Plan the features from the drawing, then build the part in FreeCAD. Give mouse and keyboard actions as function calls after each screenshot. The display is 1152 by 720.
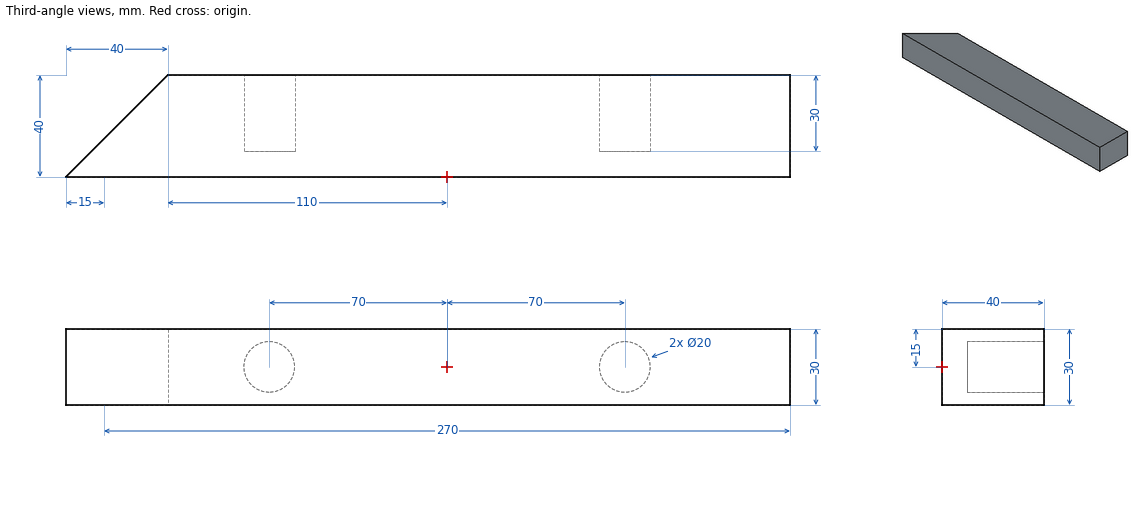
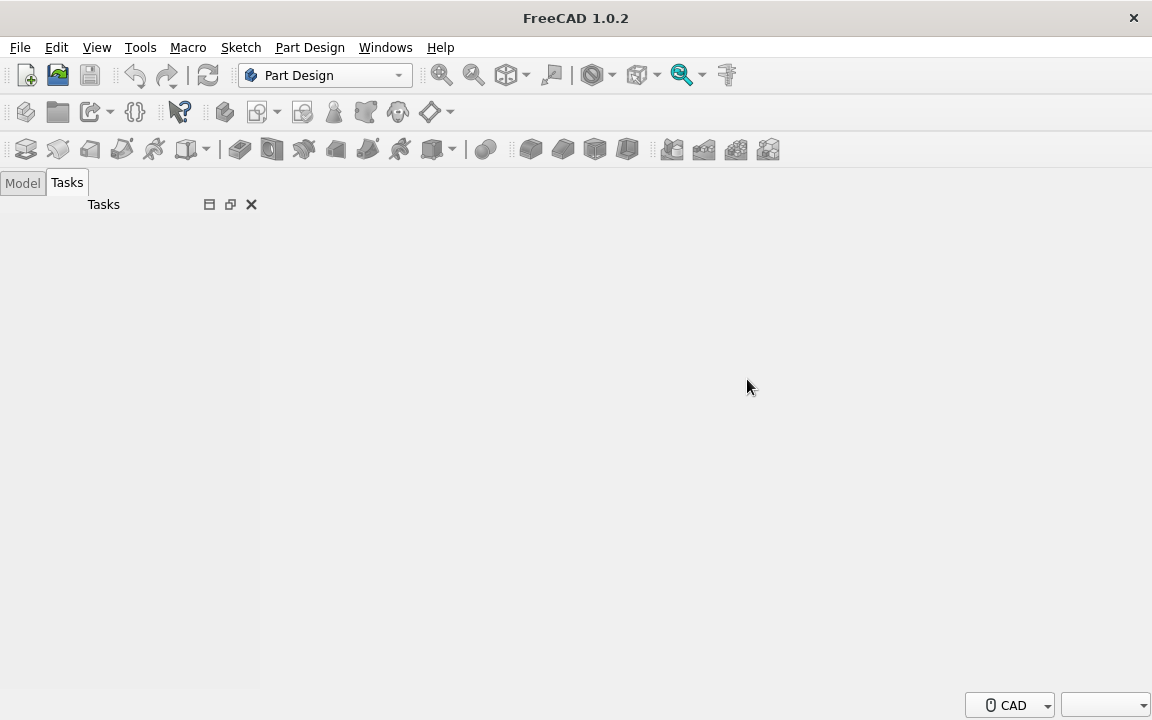
key(ctrl+n)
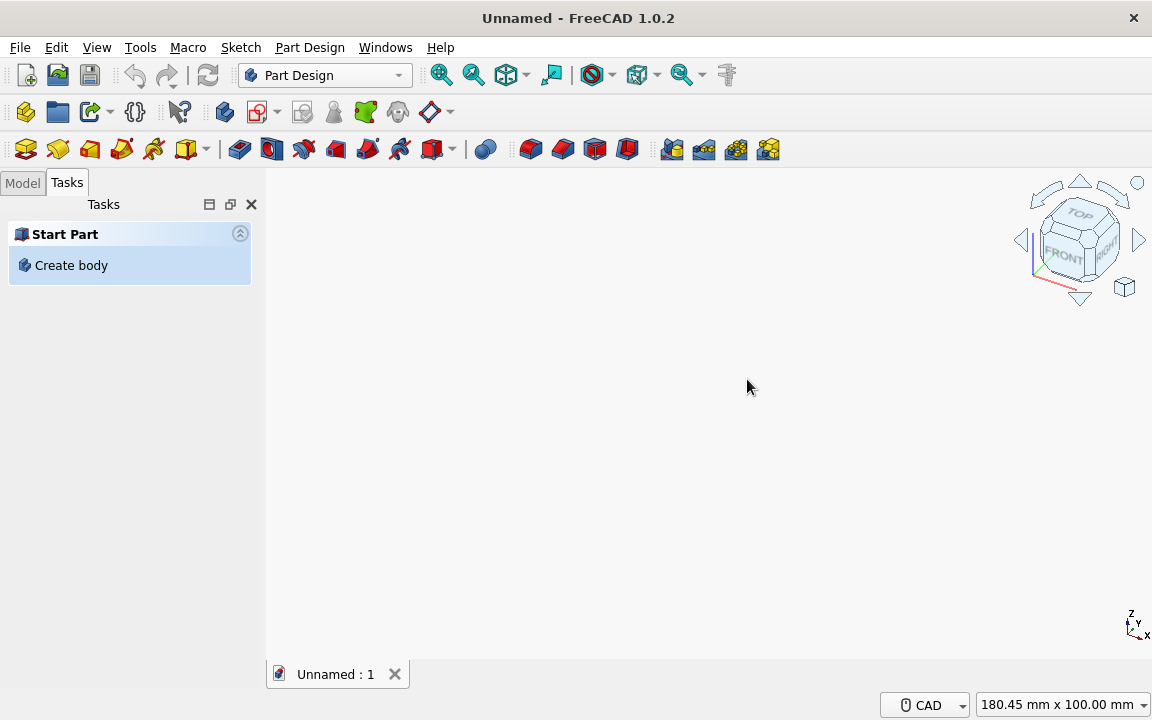
click(258, 112)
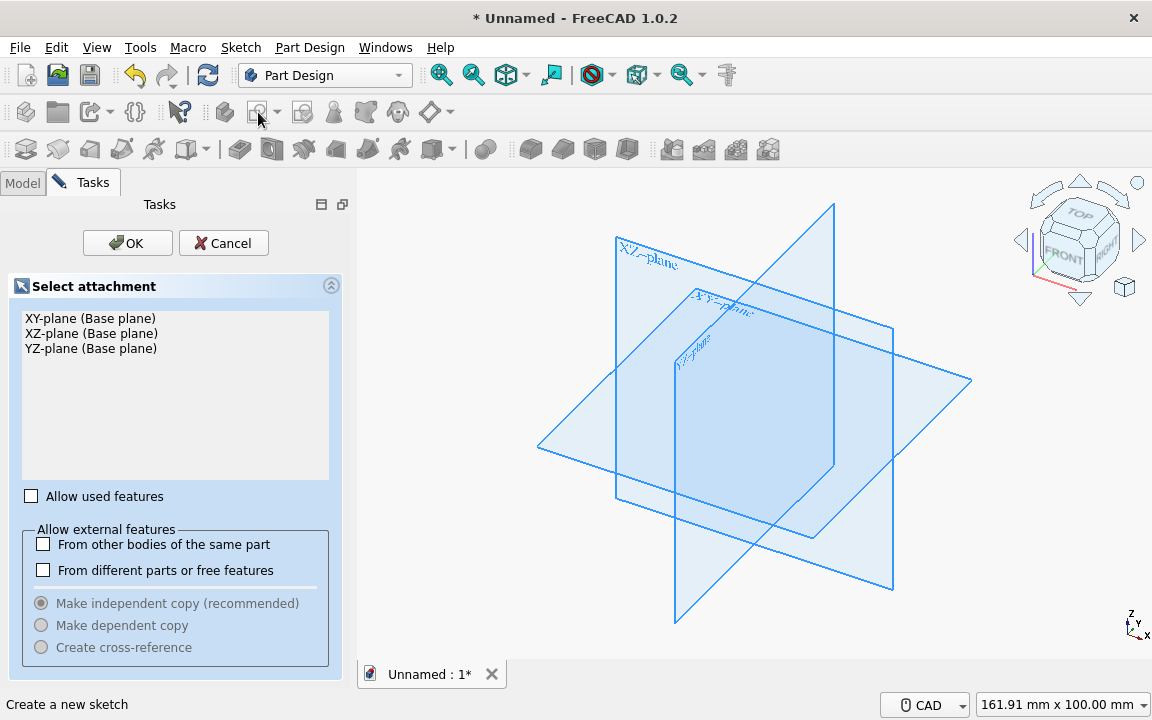
click(82, 334)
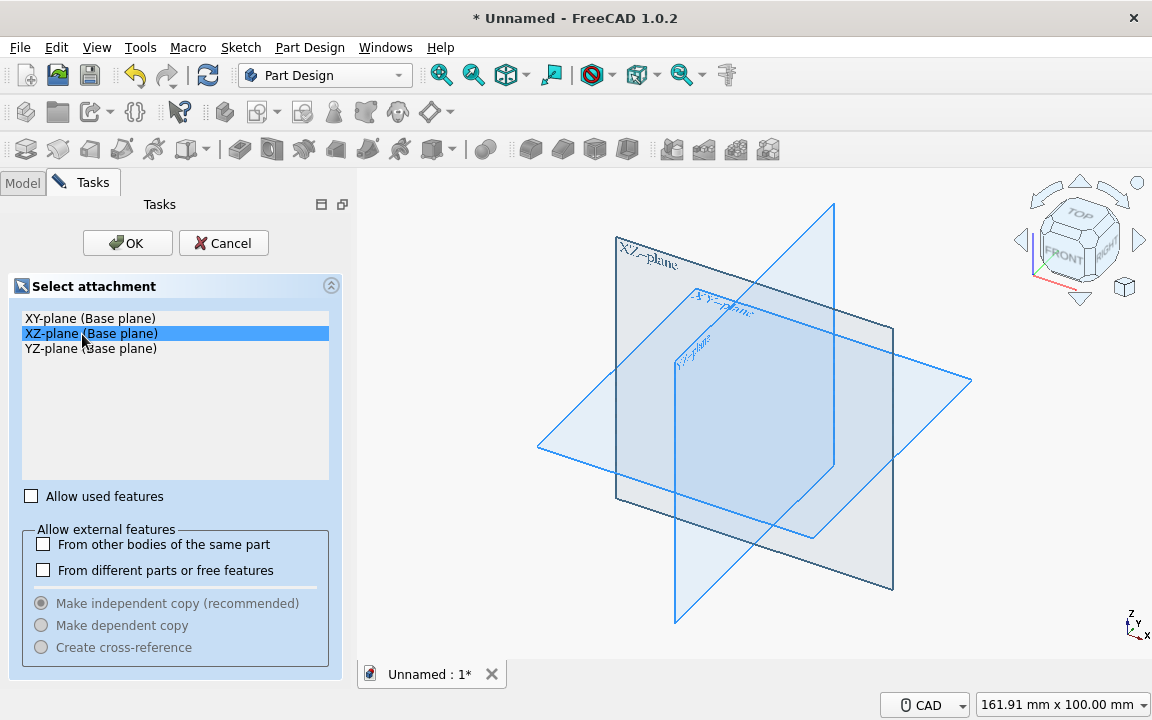
click(128, 243)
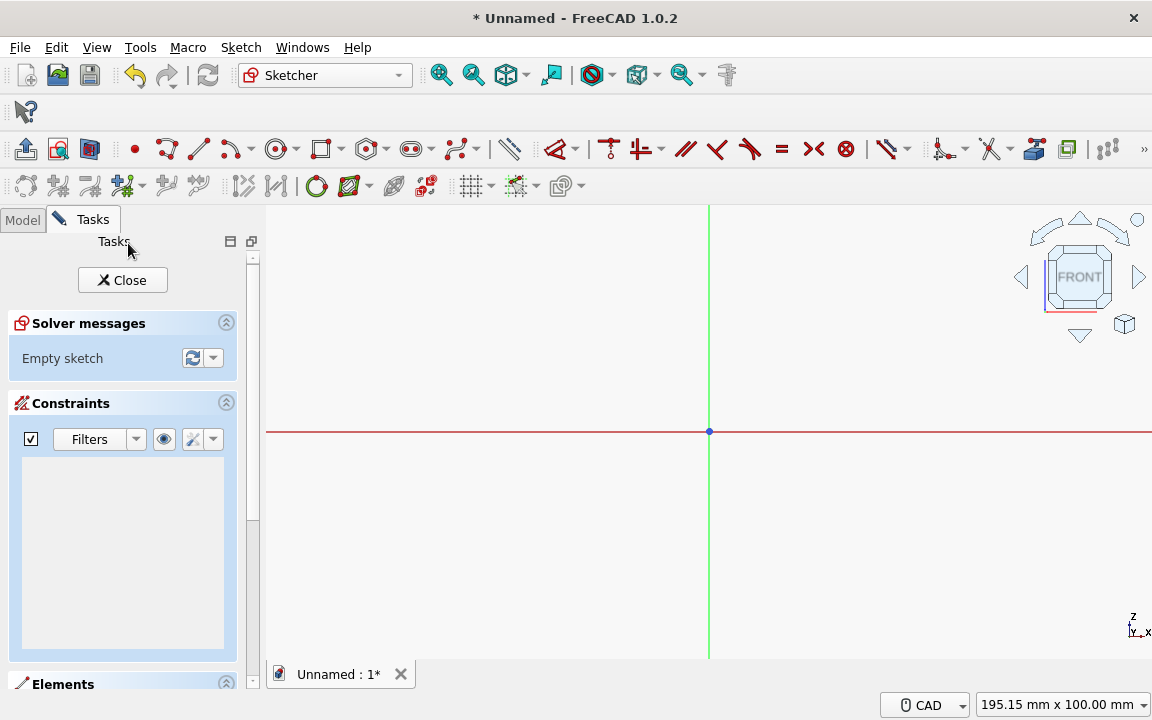
scroll(601, 432, down, 5)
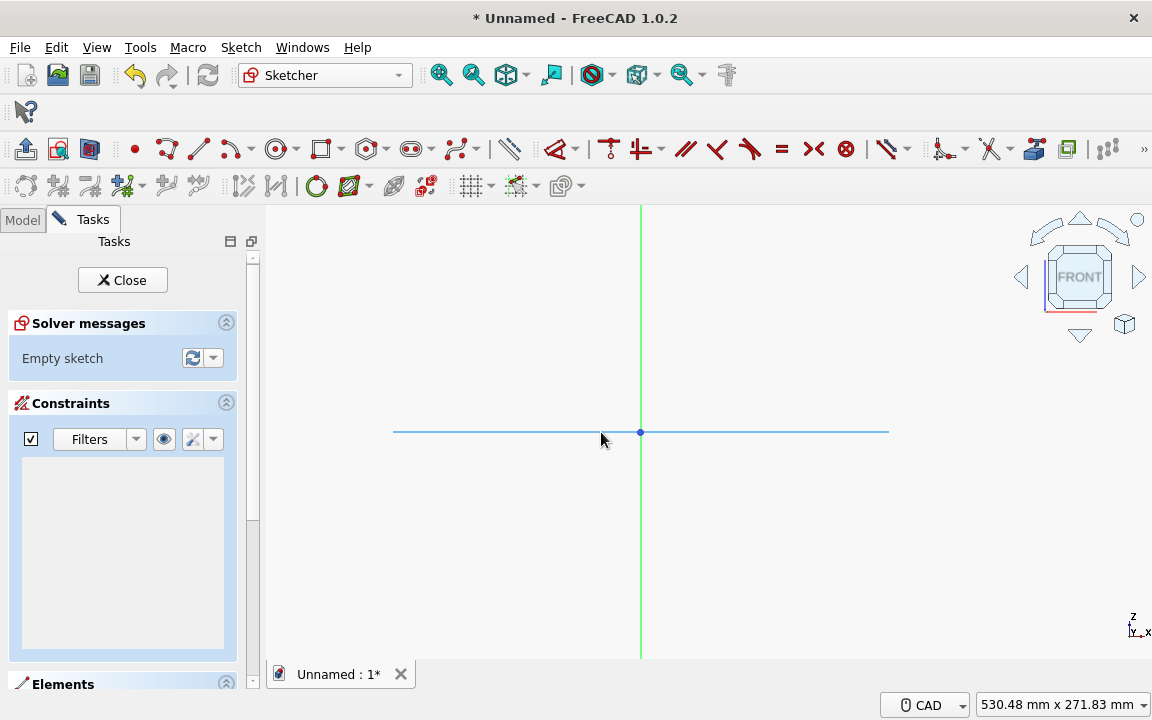
key(g)
key(v)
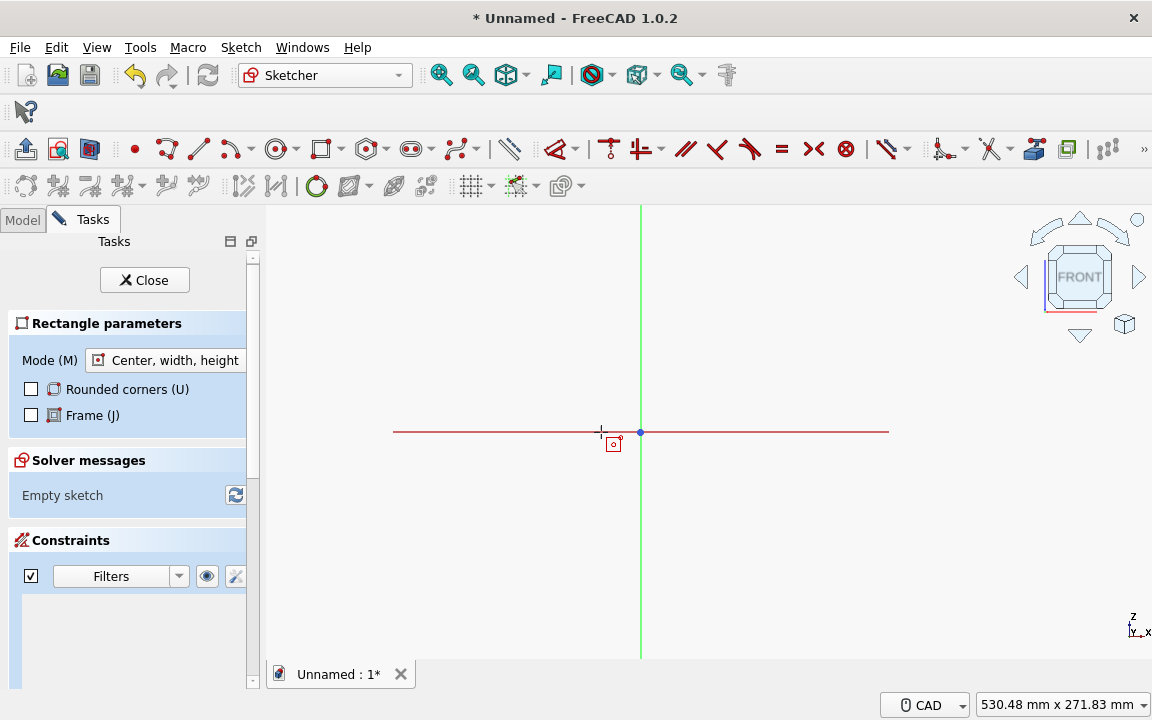
click(641, 432)
move(866, 407)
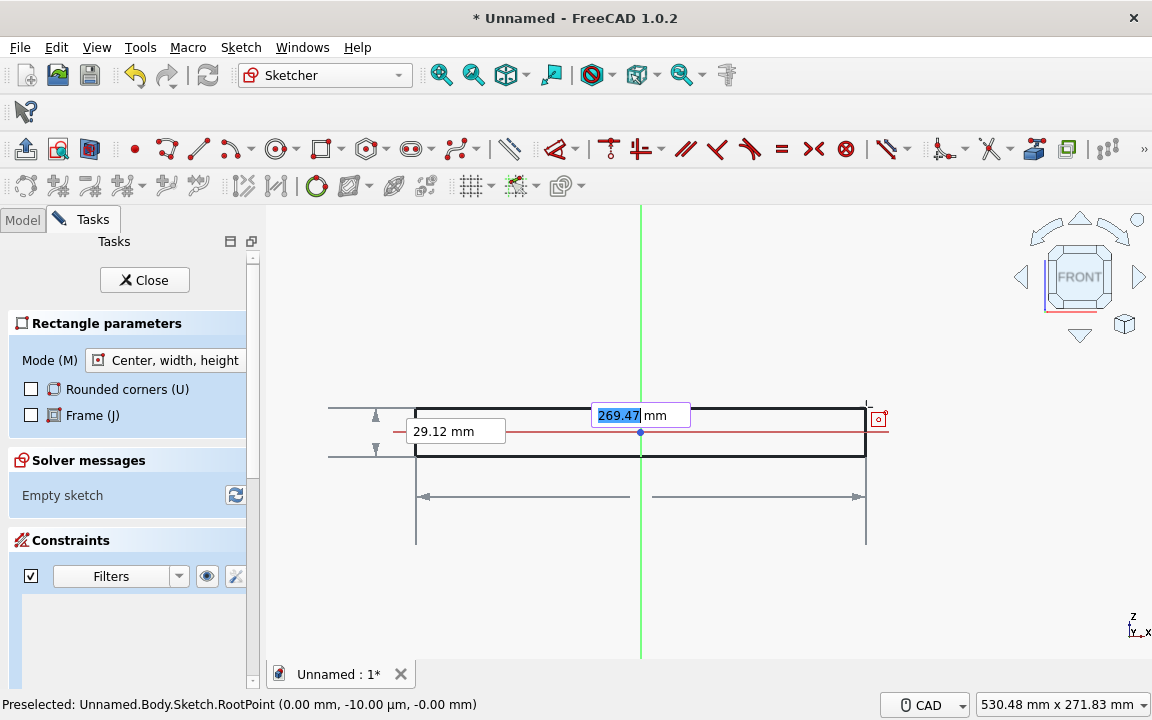
text(270)
key(Tab)
text(30)
key(Return)
key(Escape)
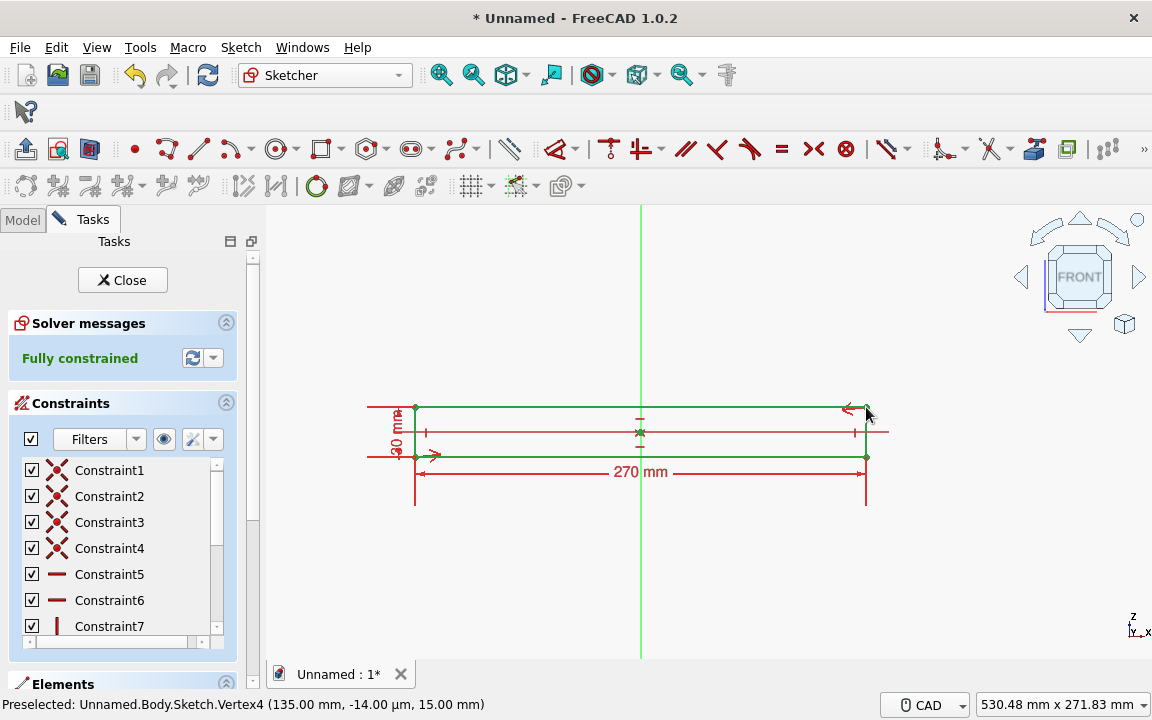
click(123, 280)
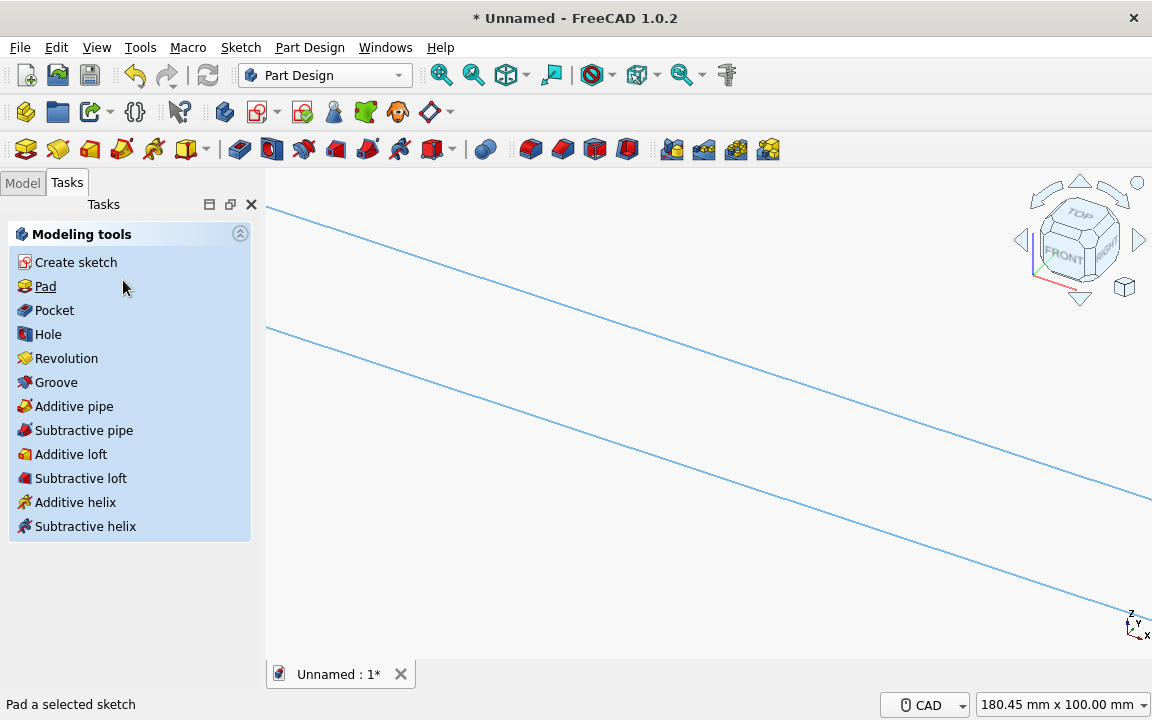
click(26, 150)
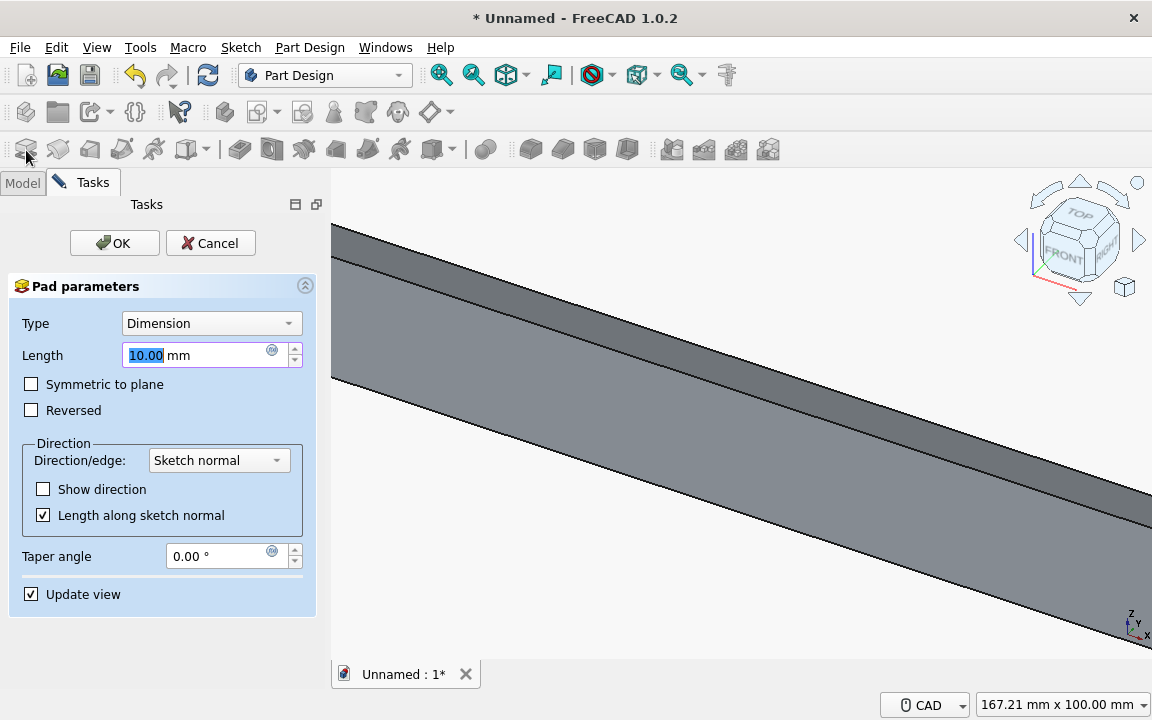
text(40)
key(Tab)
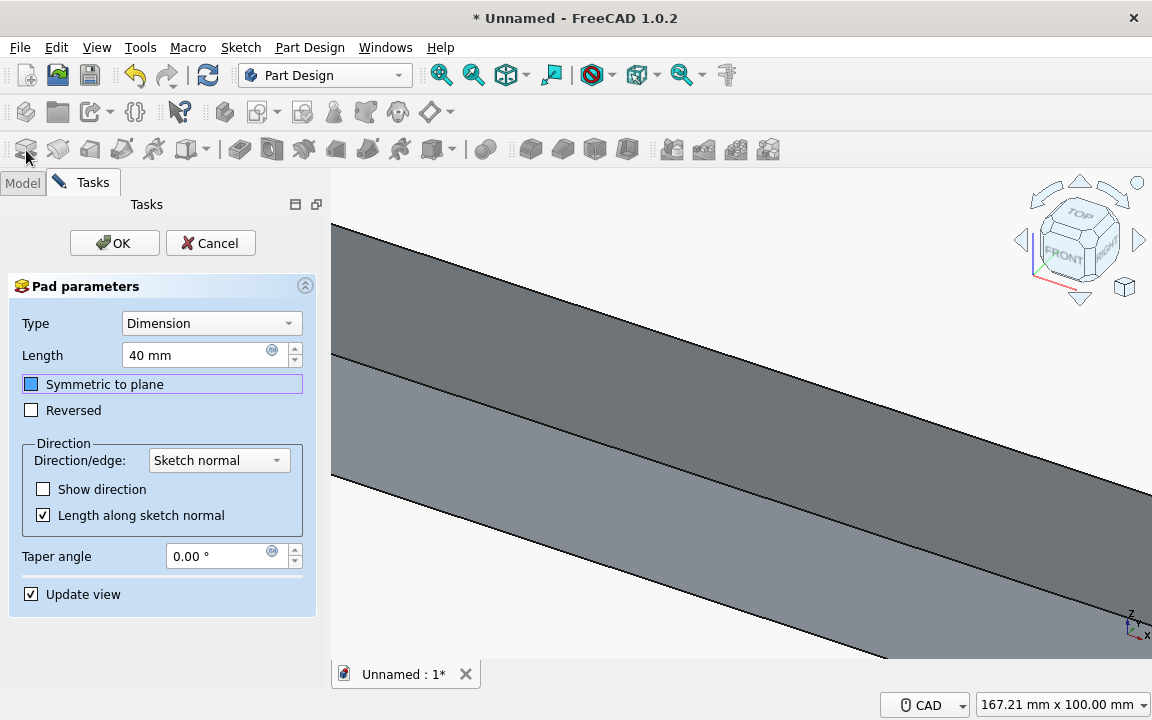
click(30, 410)